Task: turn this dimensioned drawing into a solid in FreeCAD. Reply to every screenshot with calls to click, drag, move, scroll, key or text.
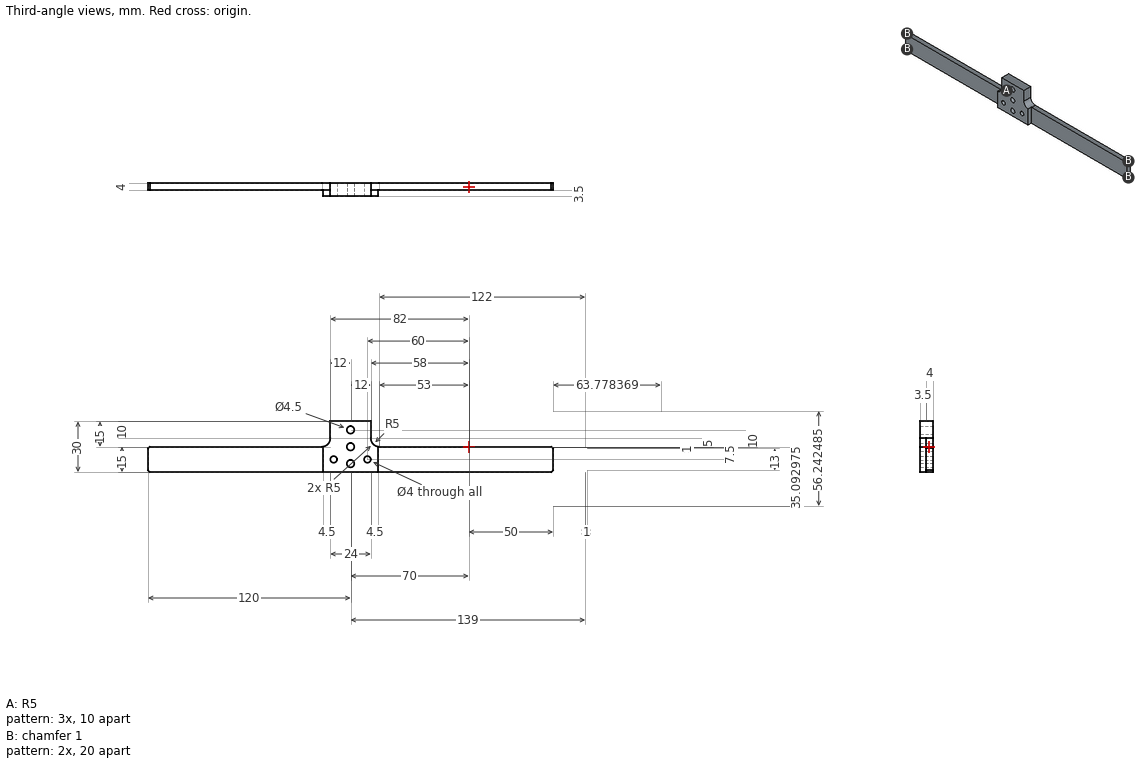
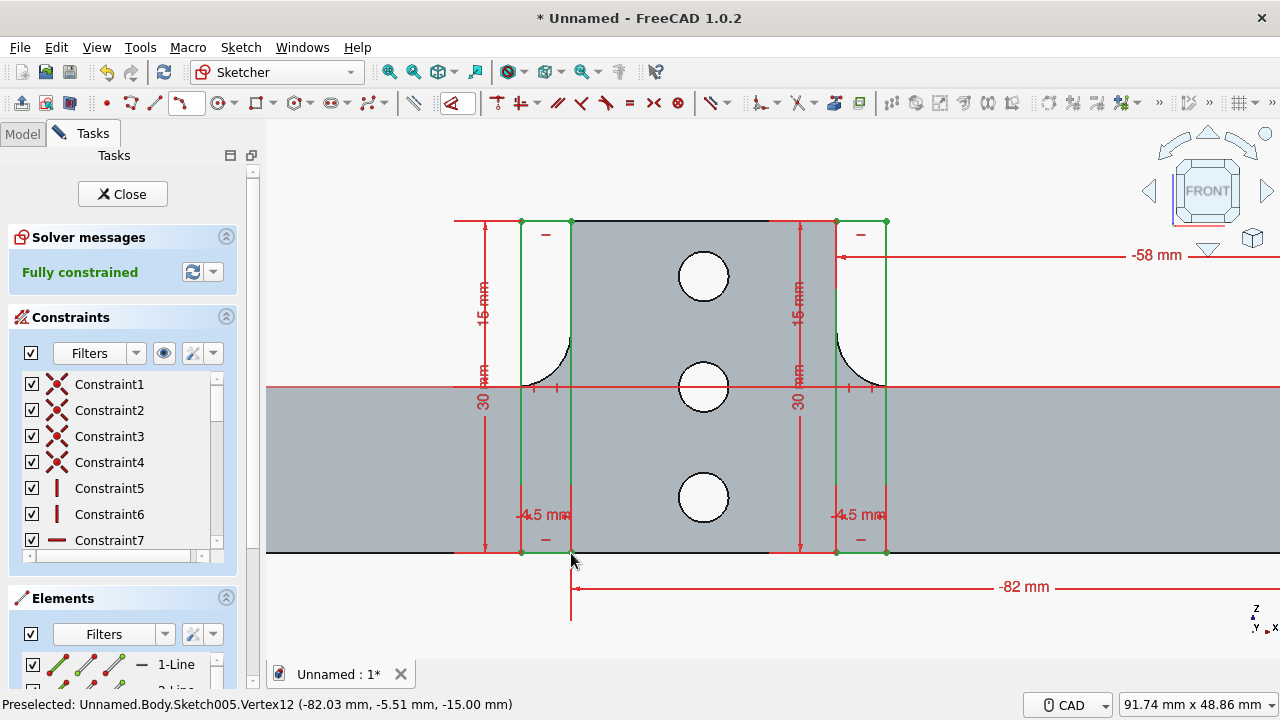
click(123, 194)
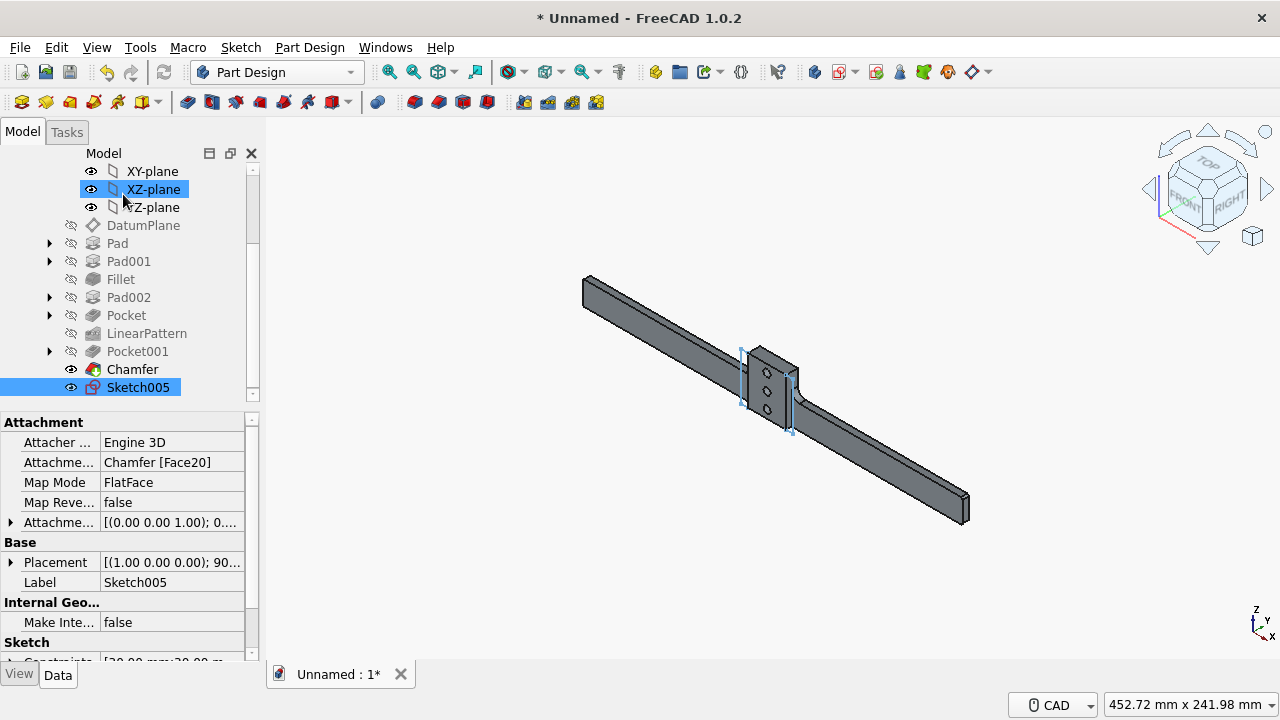
click(22, 102)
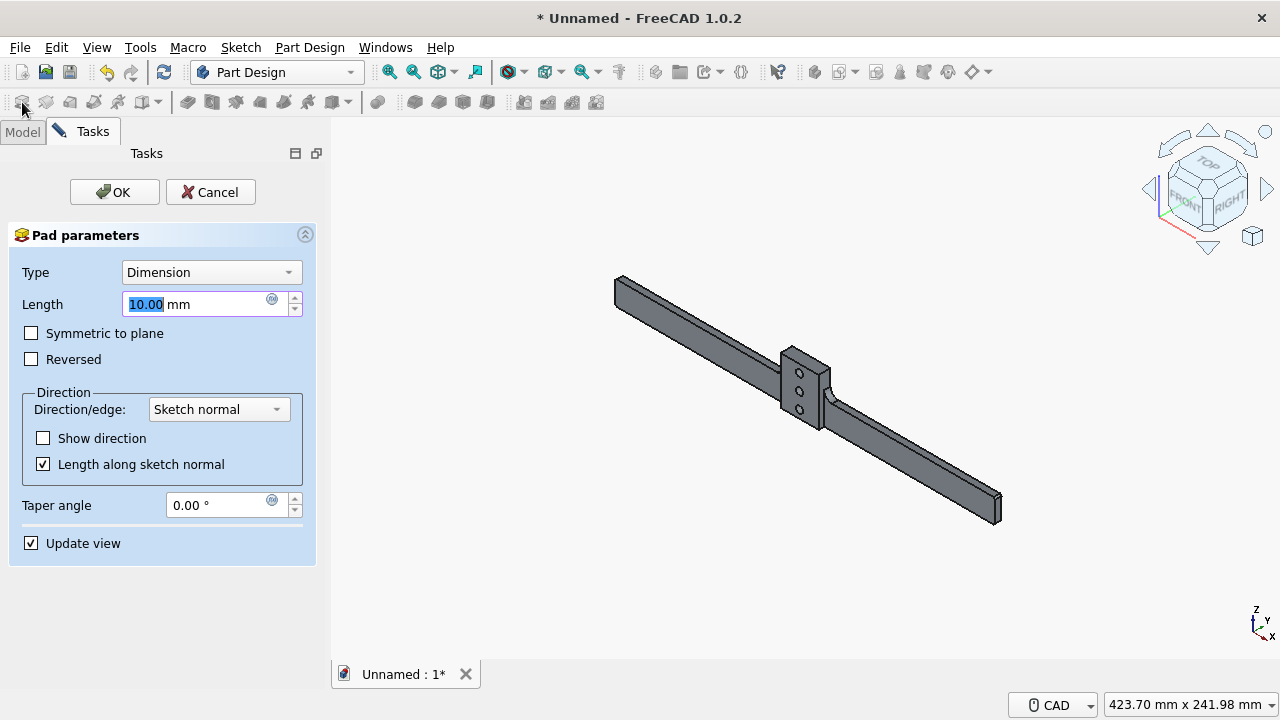
text(3.5)
key(Tab)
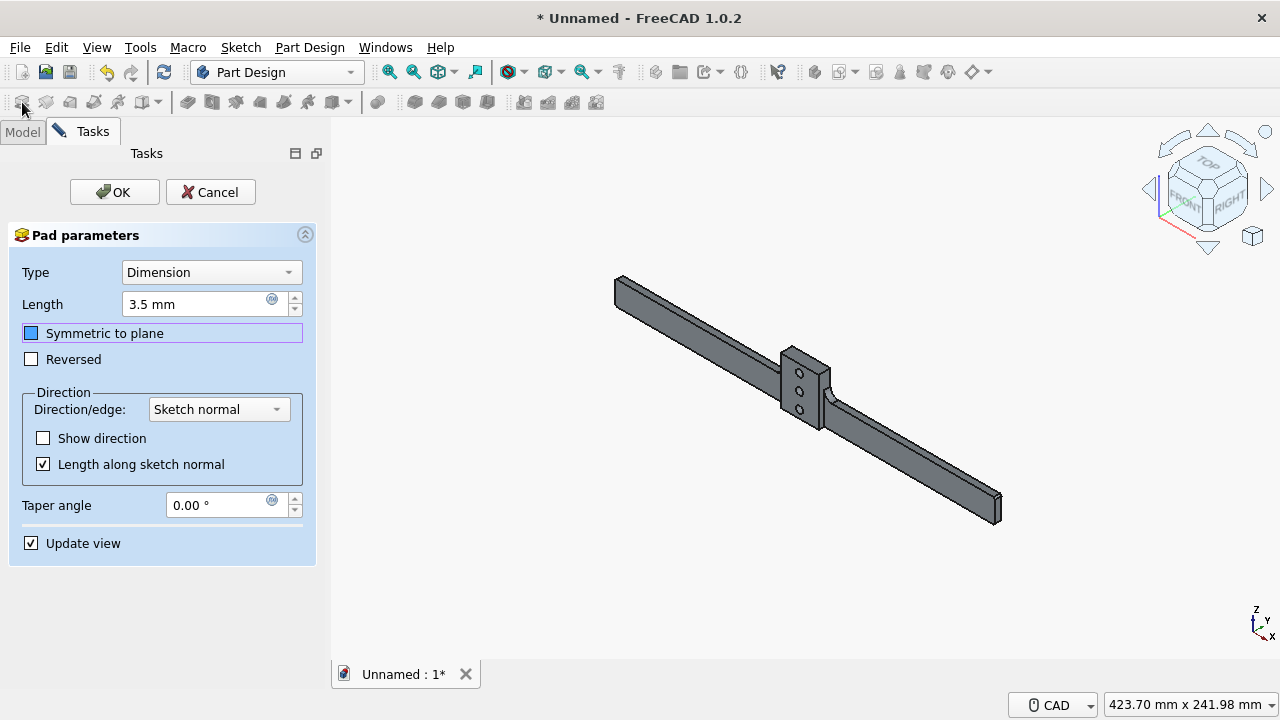
click(30, 359)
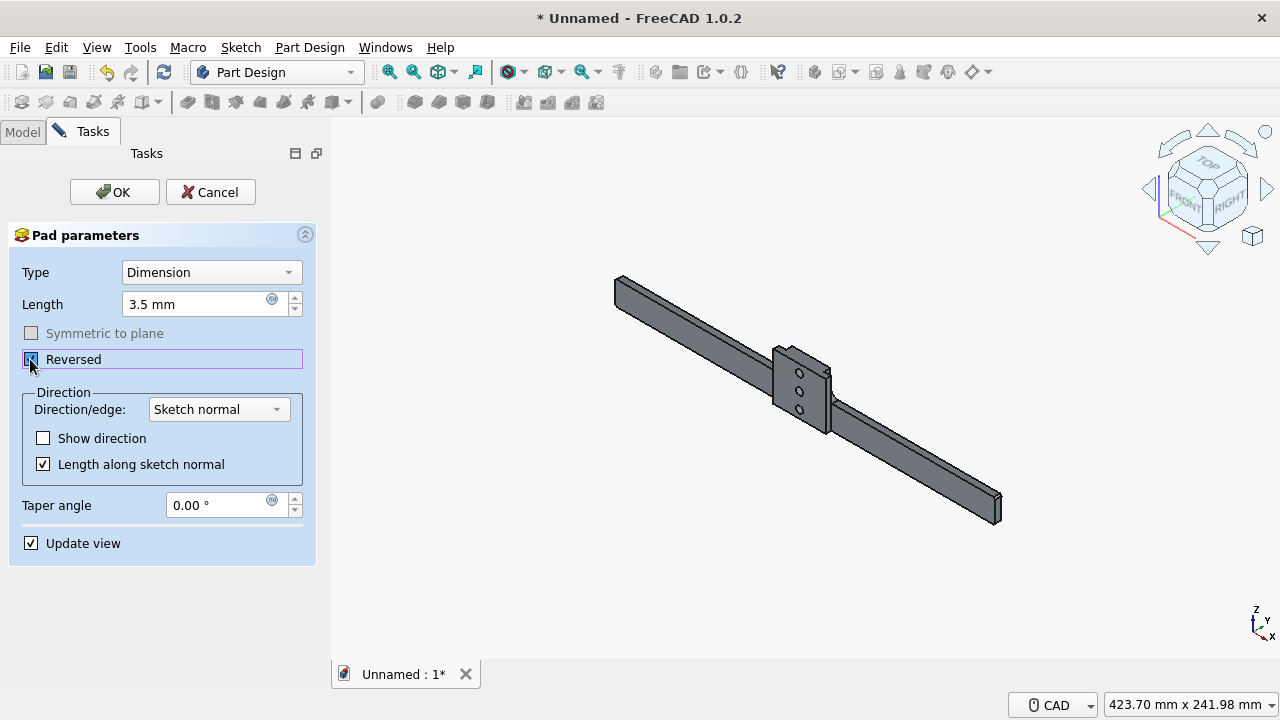
click(115, 192)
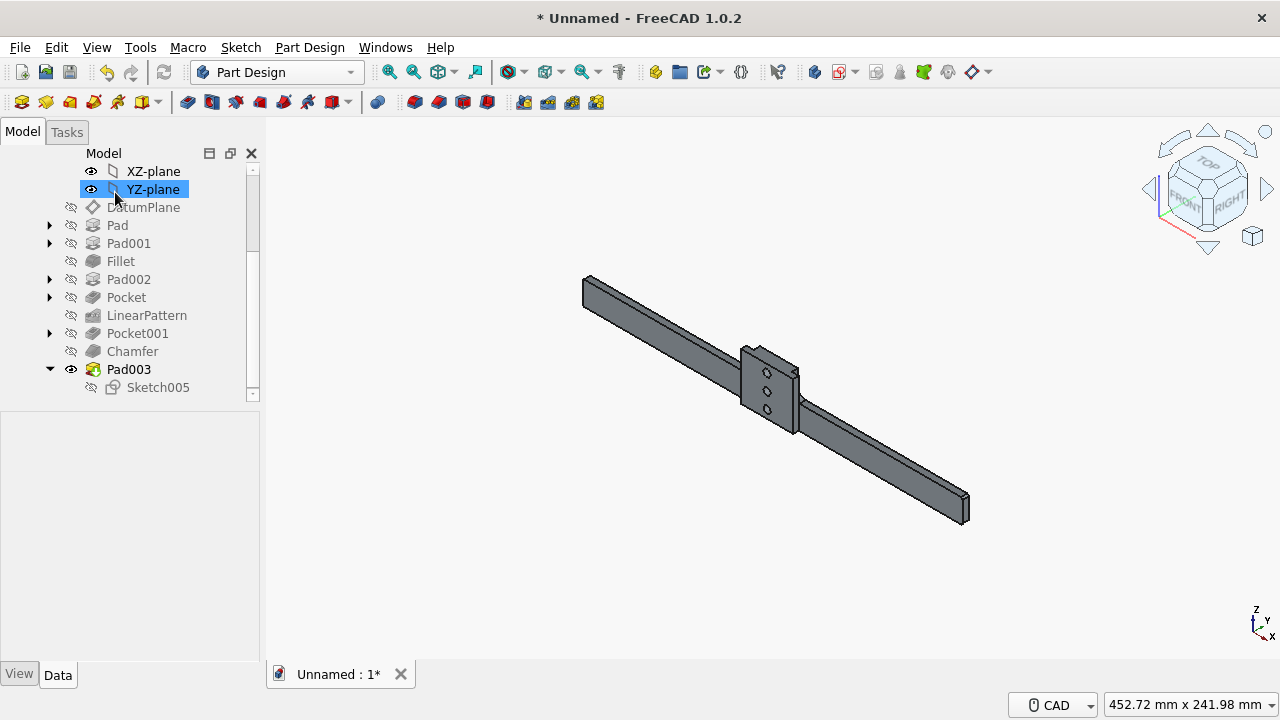
scroll(160, 275, down, 3)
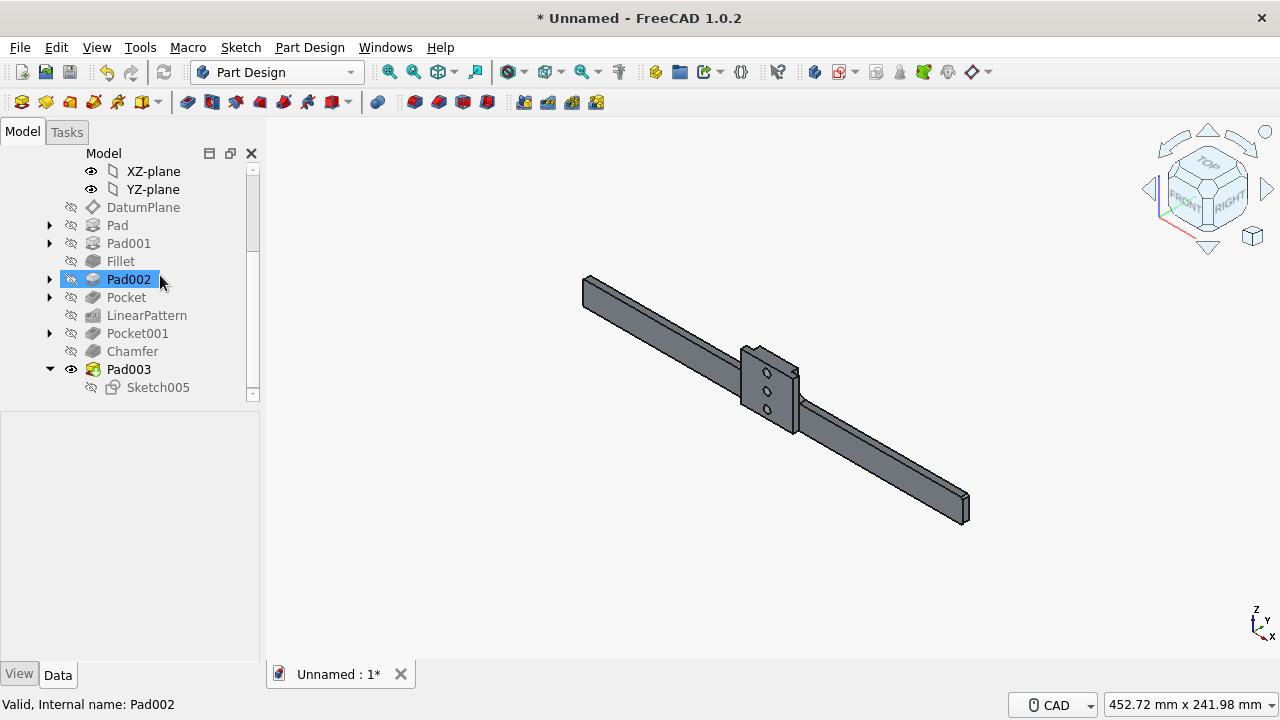
scroll(160, 275, up, 15)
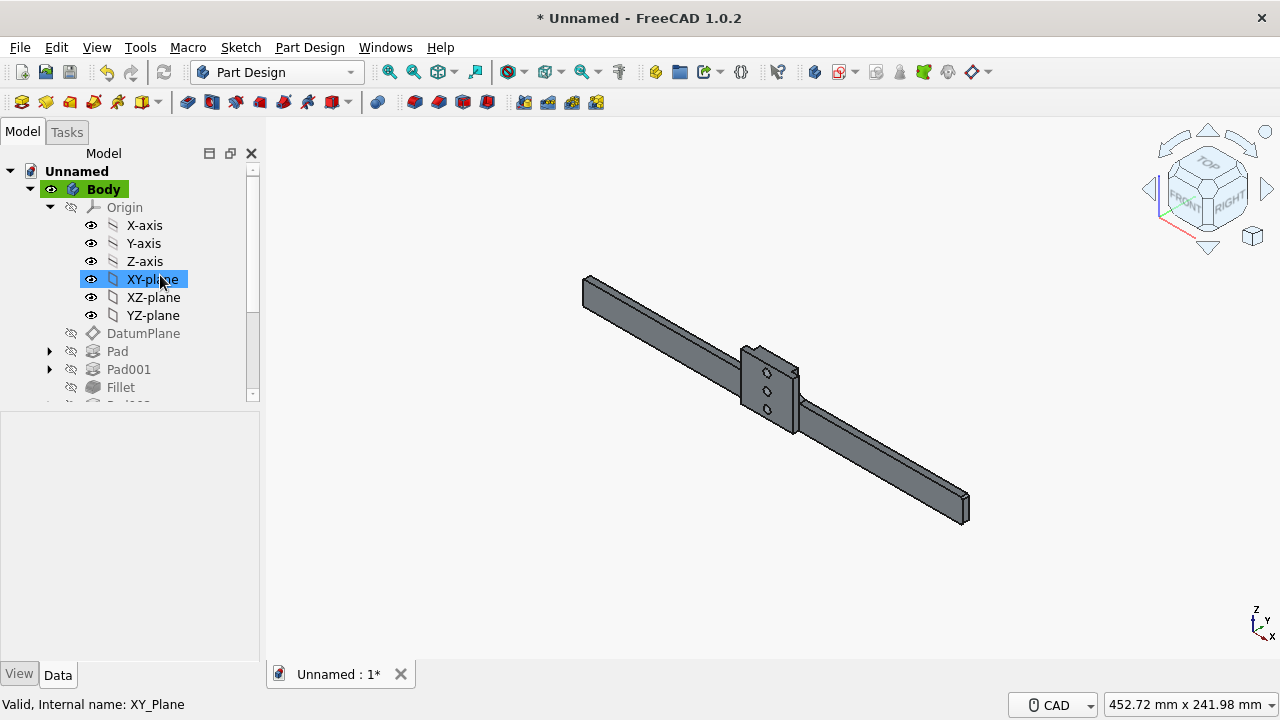
click(136, 297)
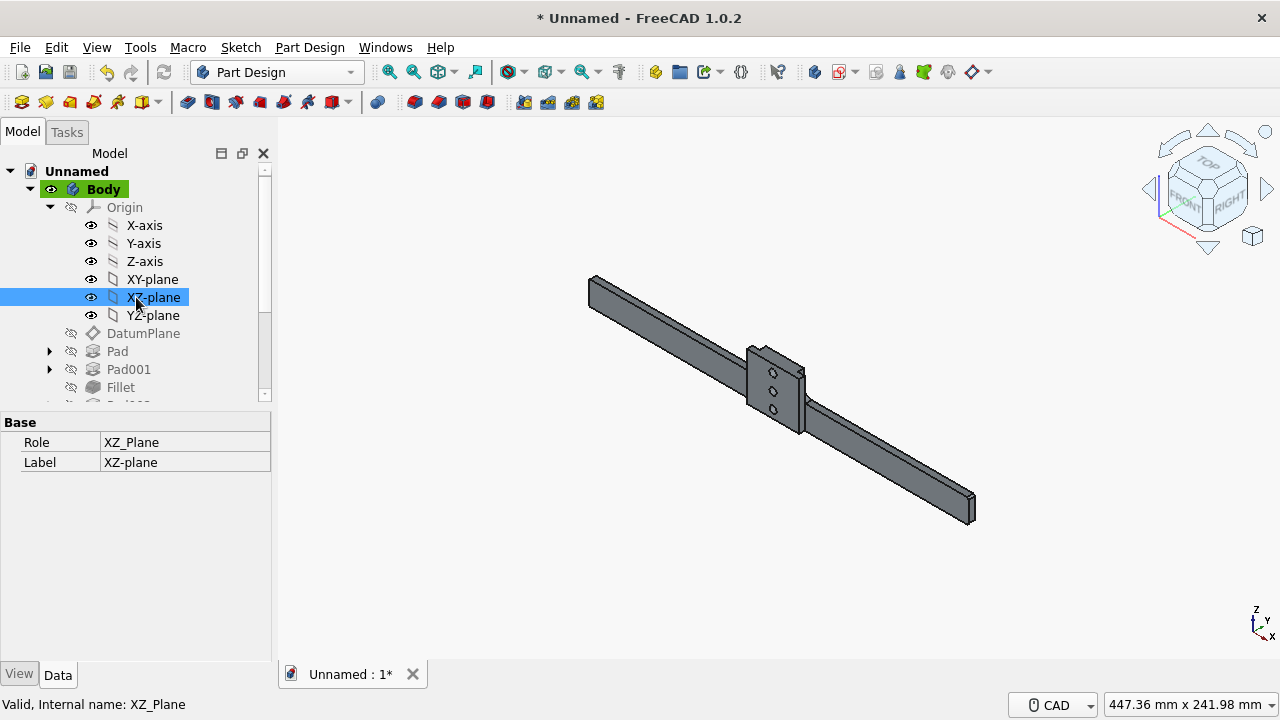
click(972, 72)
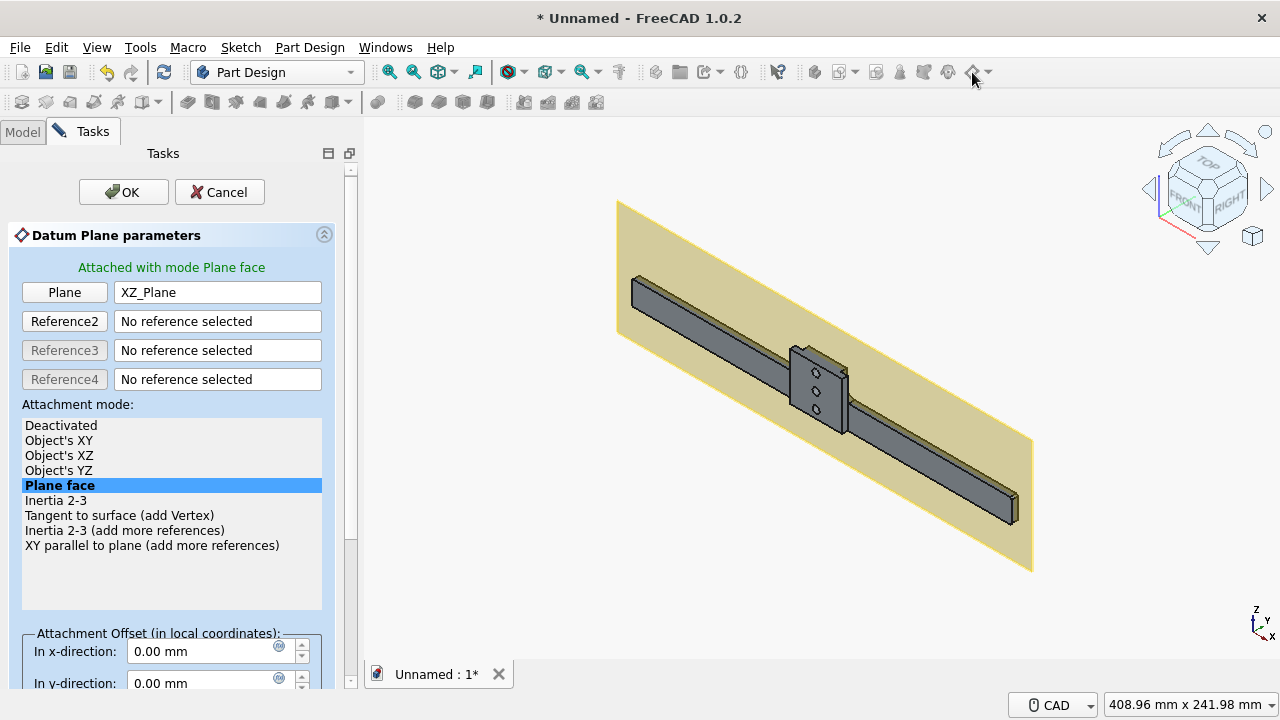
scroll(351, 426, down, 2)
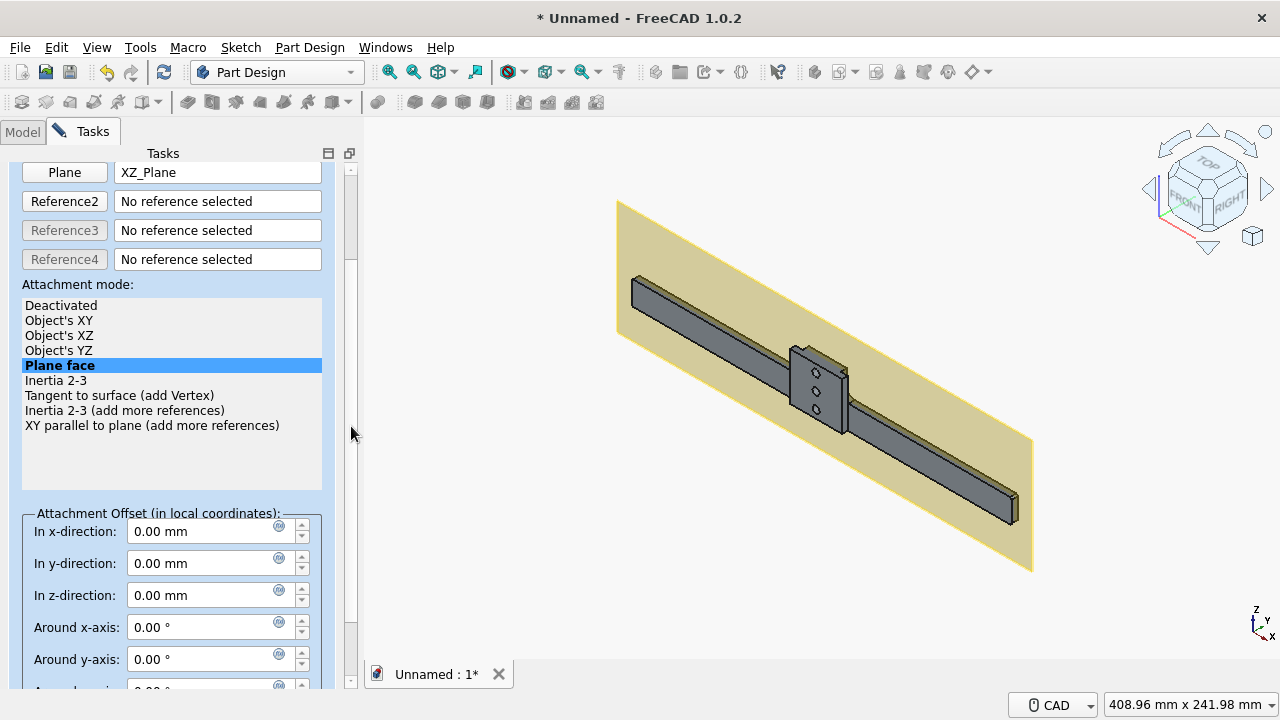
triple_click(210, 595)